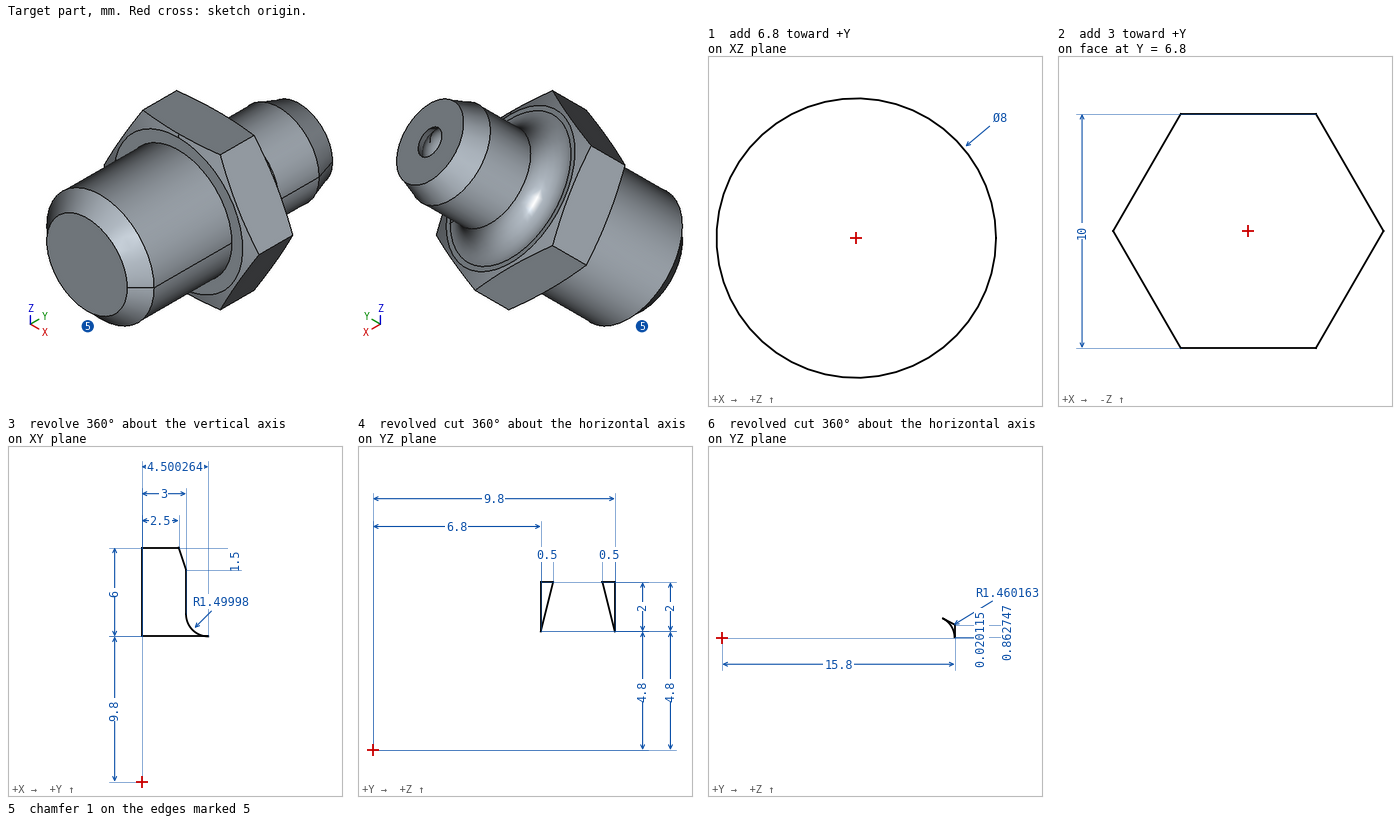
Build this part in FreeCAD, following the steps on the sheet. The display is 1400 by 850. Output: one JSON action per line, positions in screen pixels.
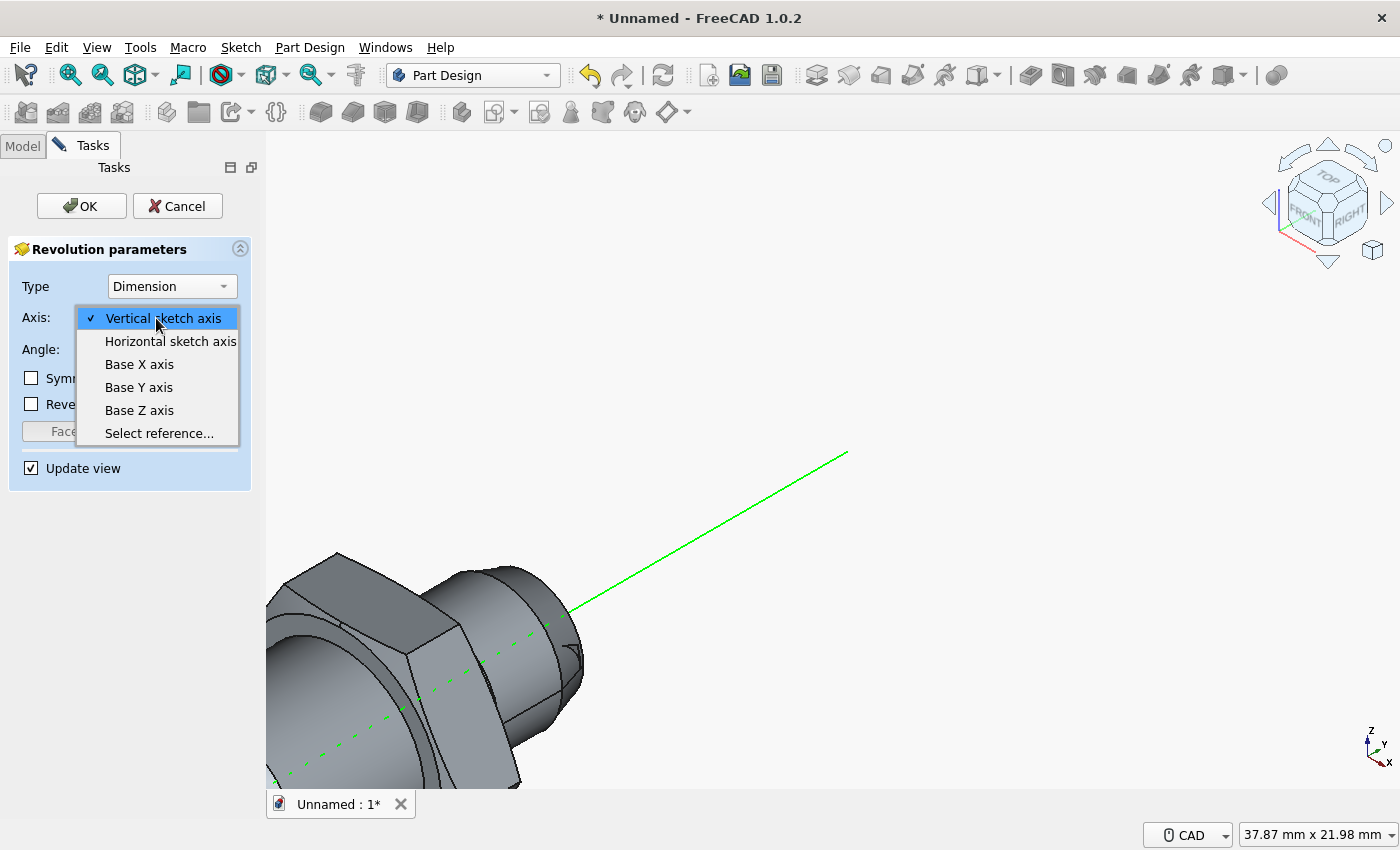
{"action": "left_click", "coordinate": [156, 342]}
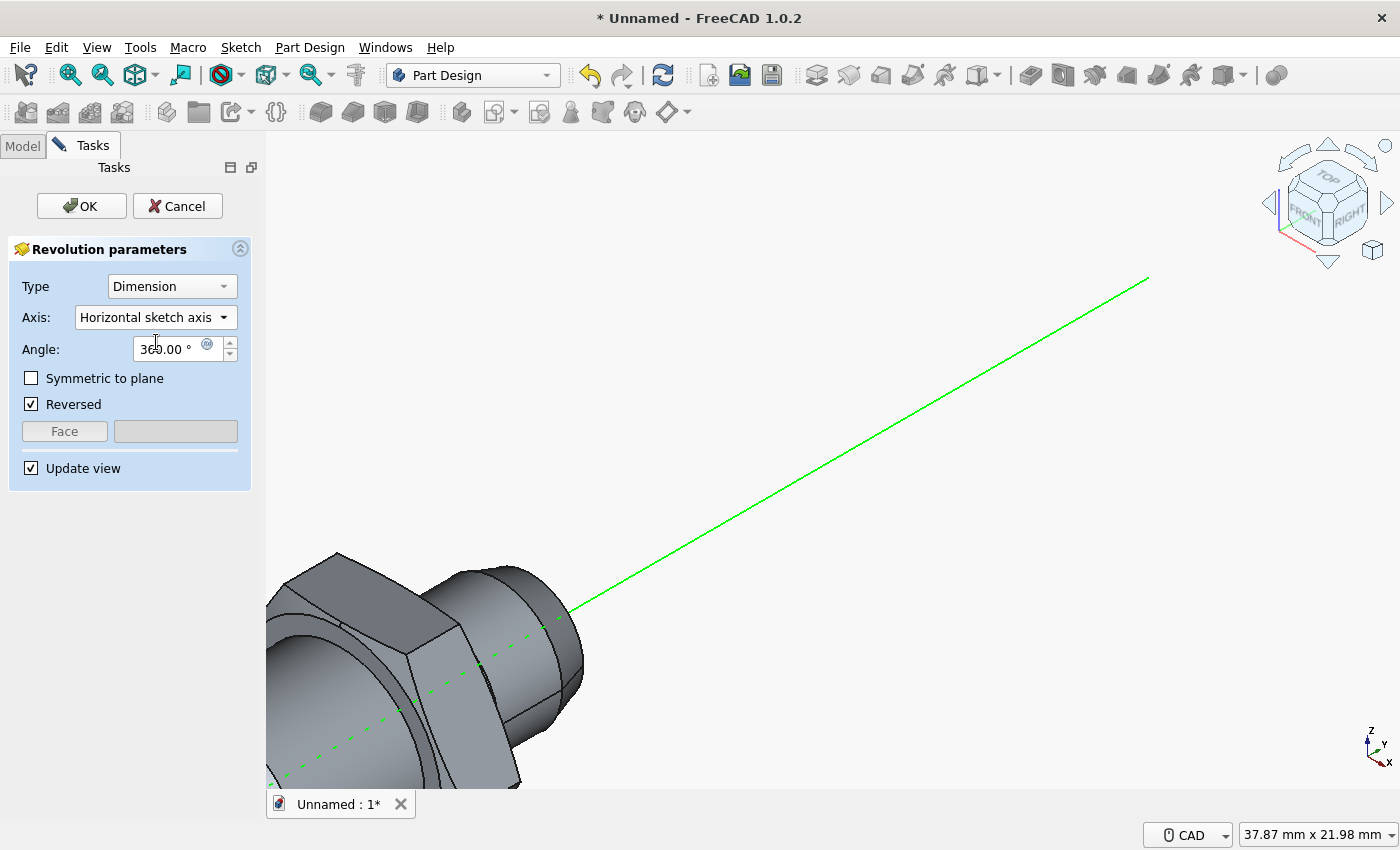
{"action": "left_click", "coordinate": [82, 206]}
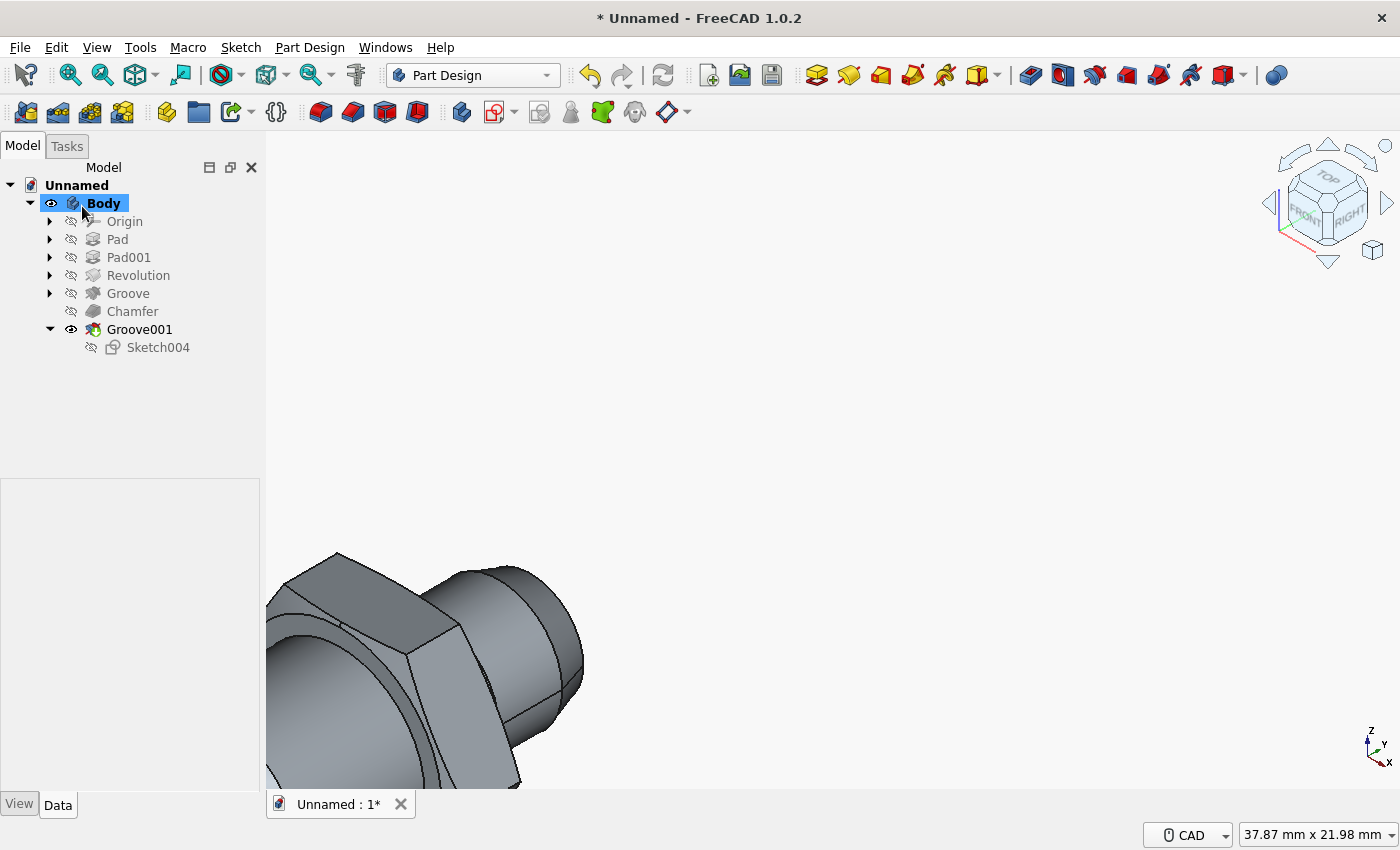
{"action": "key", "text": "v f"}